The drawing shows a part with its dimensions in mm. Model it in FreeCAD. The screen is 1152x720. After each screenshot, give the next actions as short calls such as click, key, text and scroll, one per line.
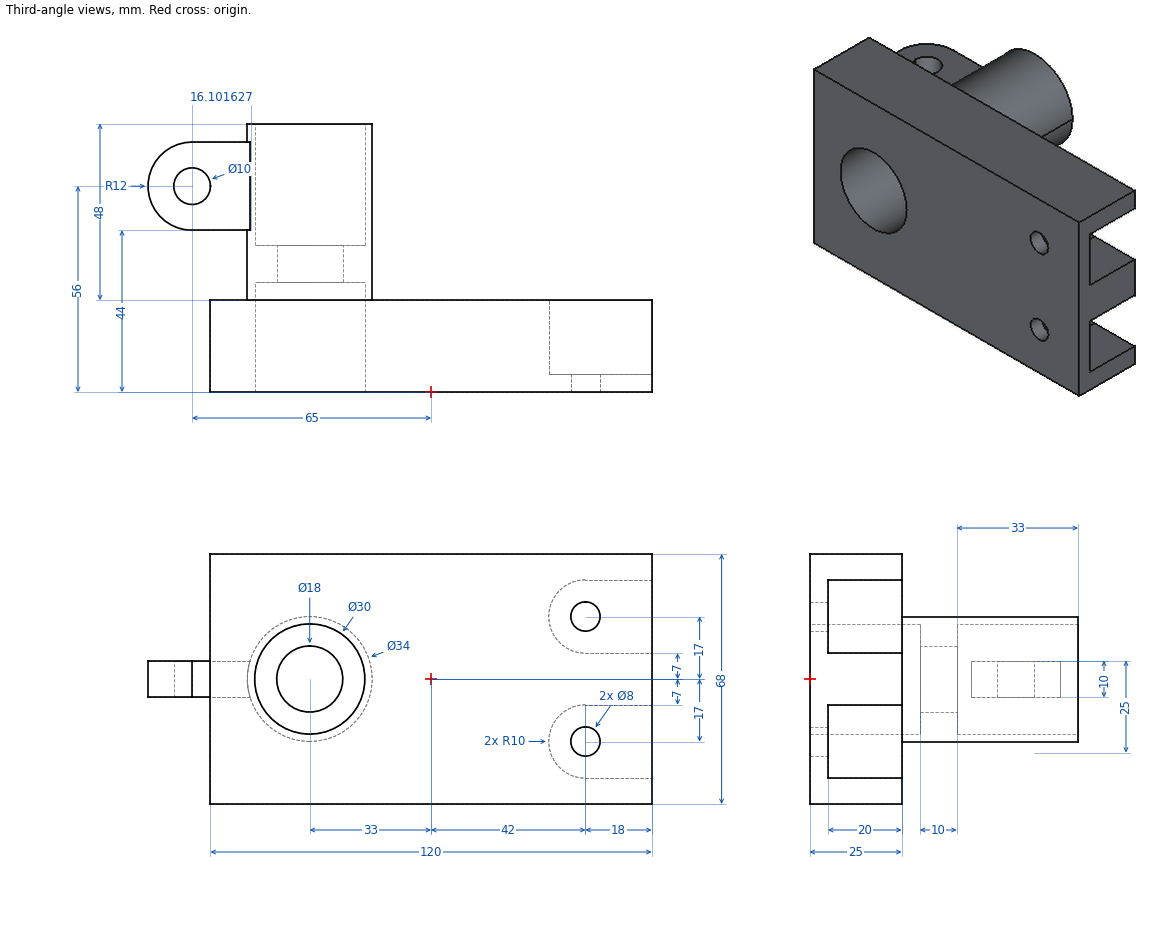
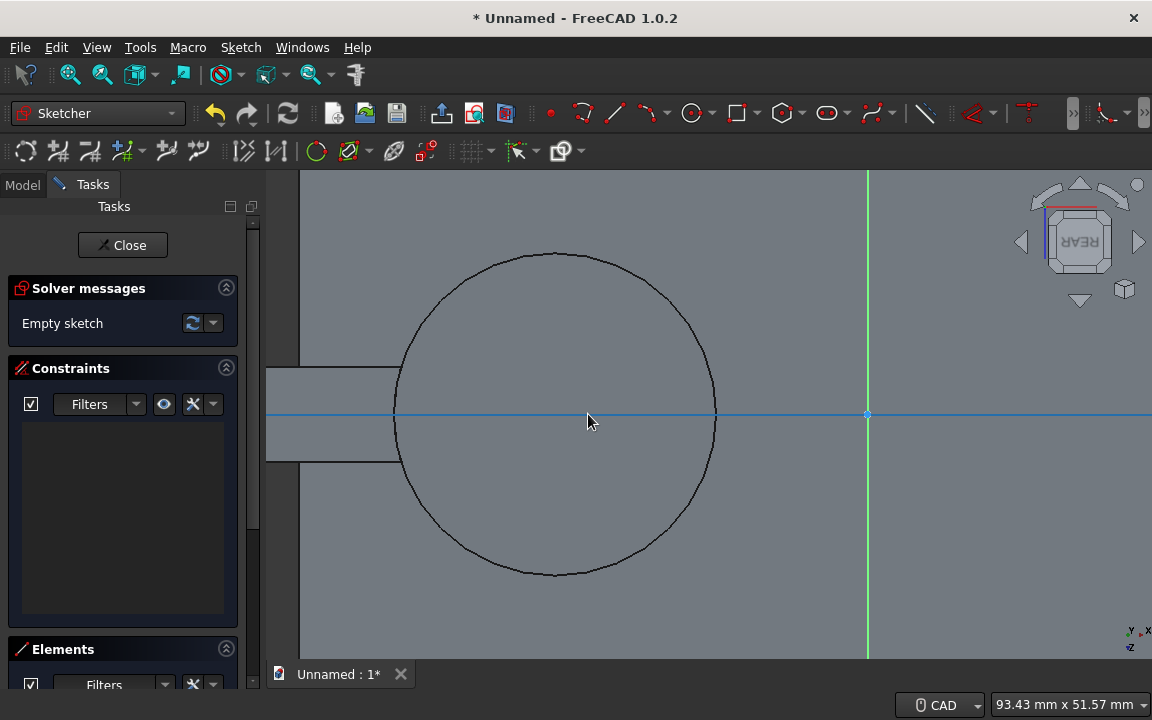
click(692, 114)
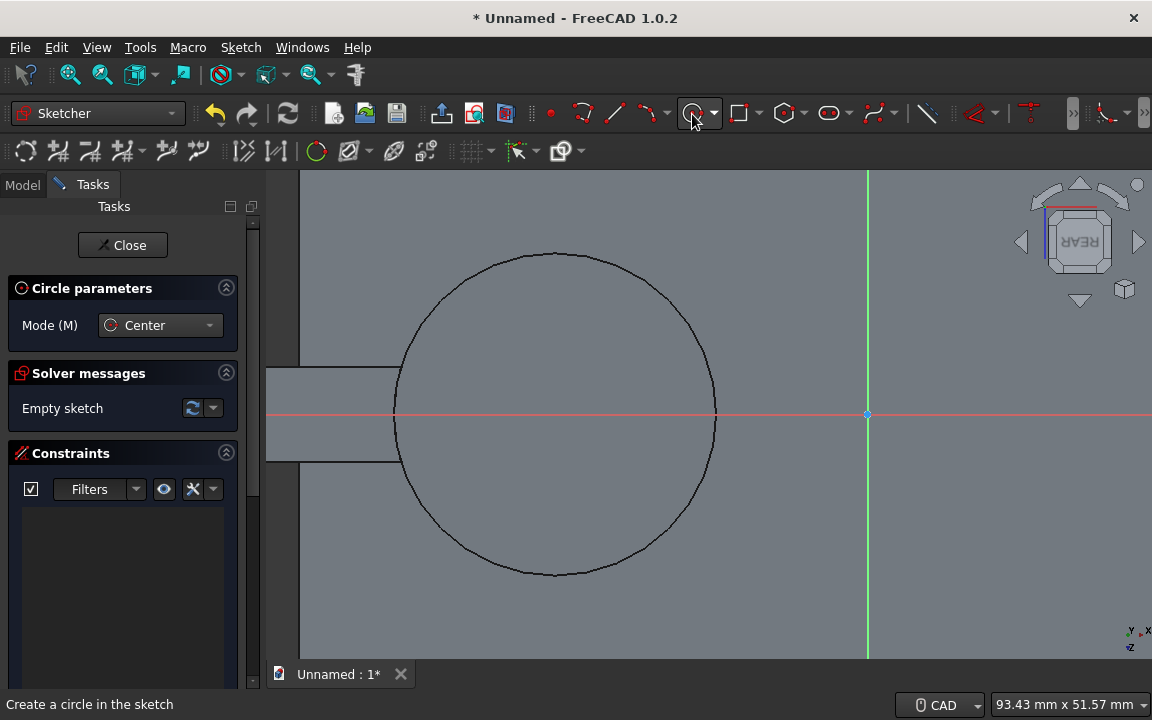
click(555, 414)
move(656, 314)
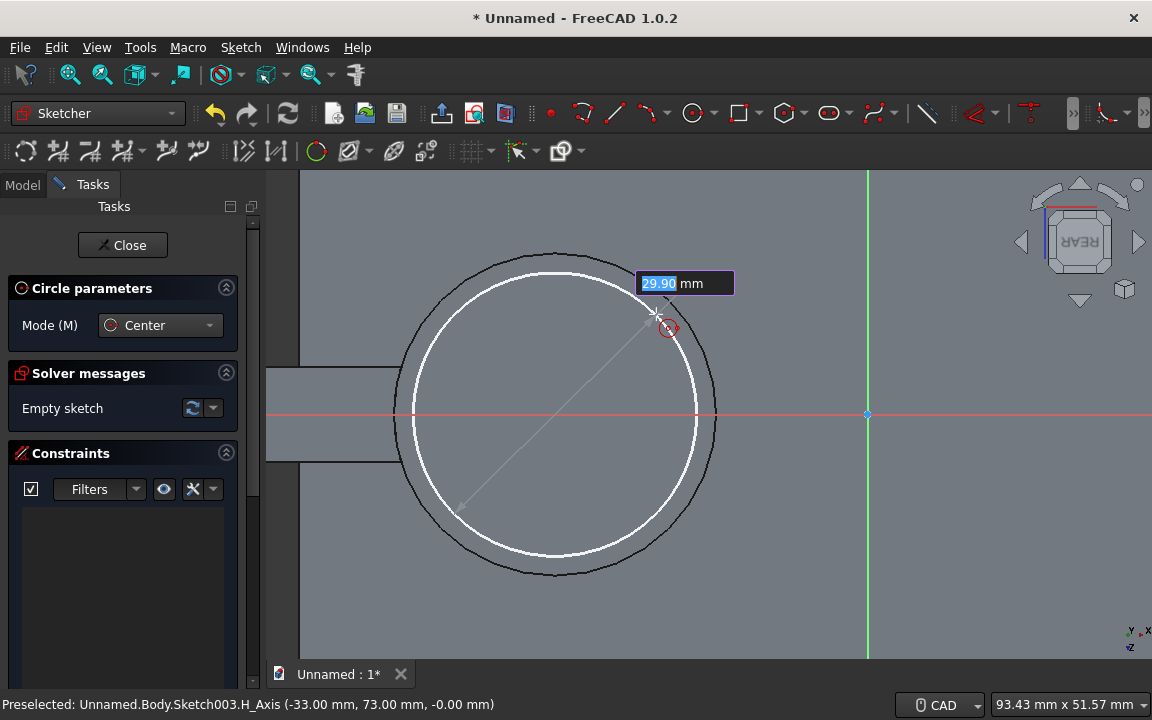
text(30)
key(Return)
key(Escape)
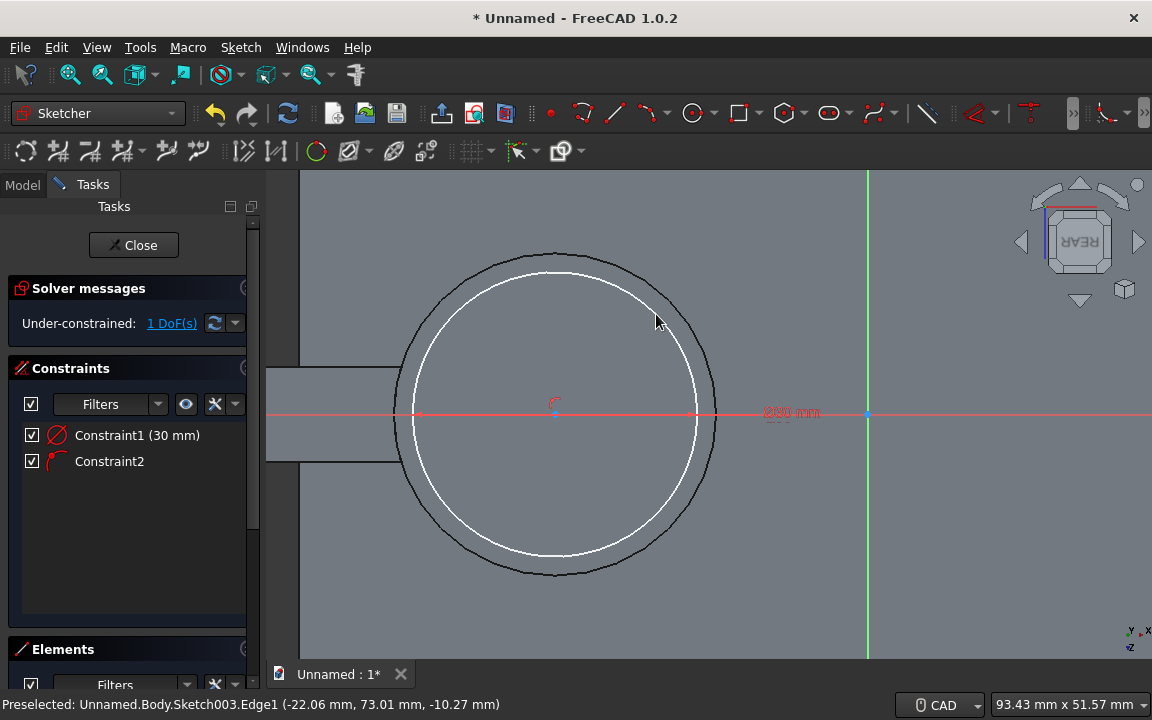
click(974, 114)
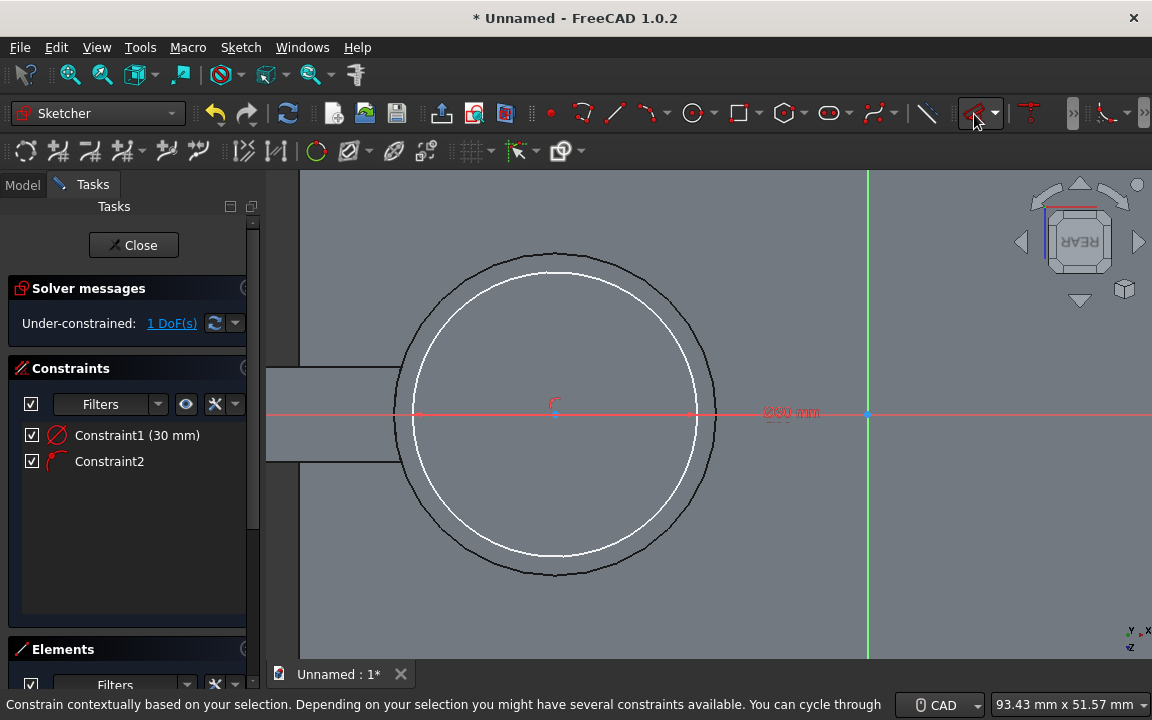
click(555, 414)
click(711, 448)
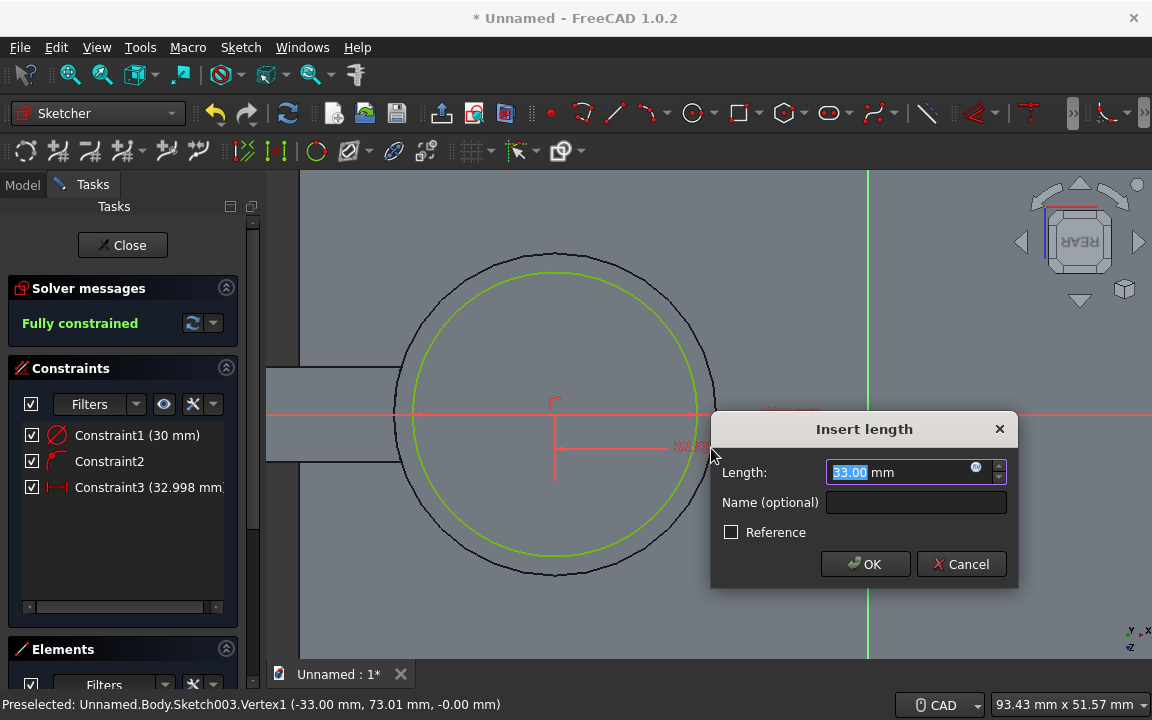
text(33)
key(Return)
key(Escape)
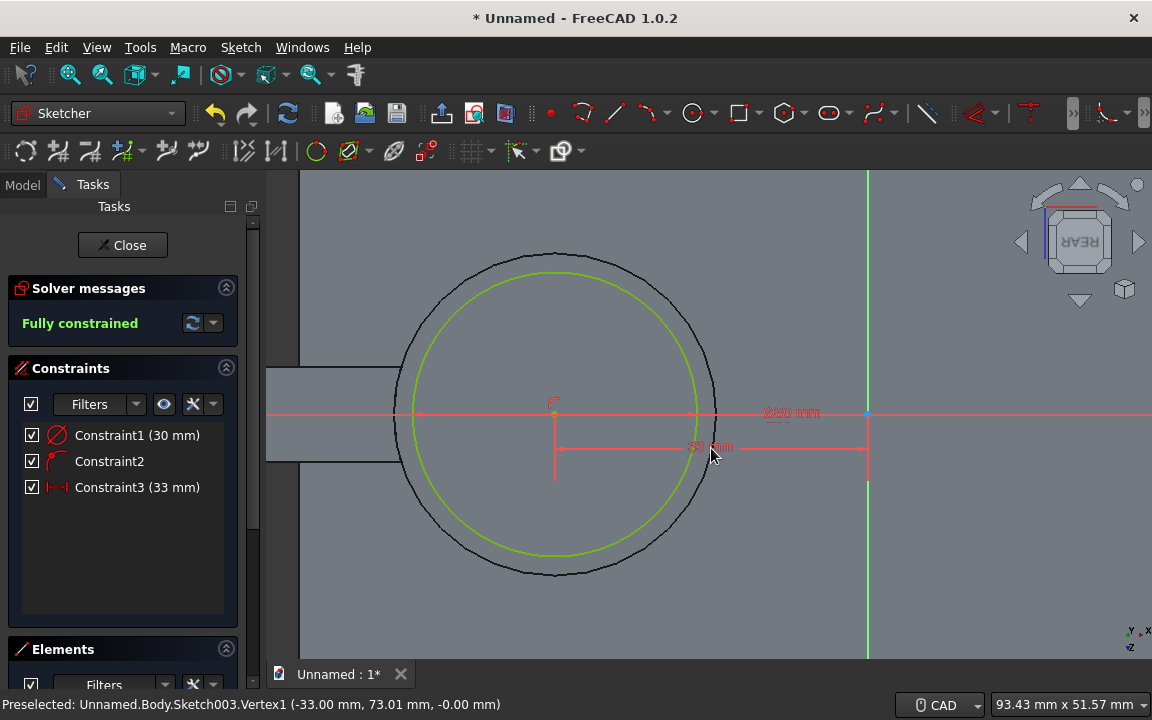
click(123, 245)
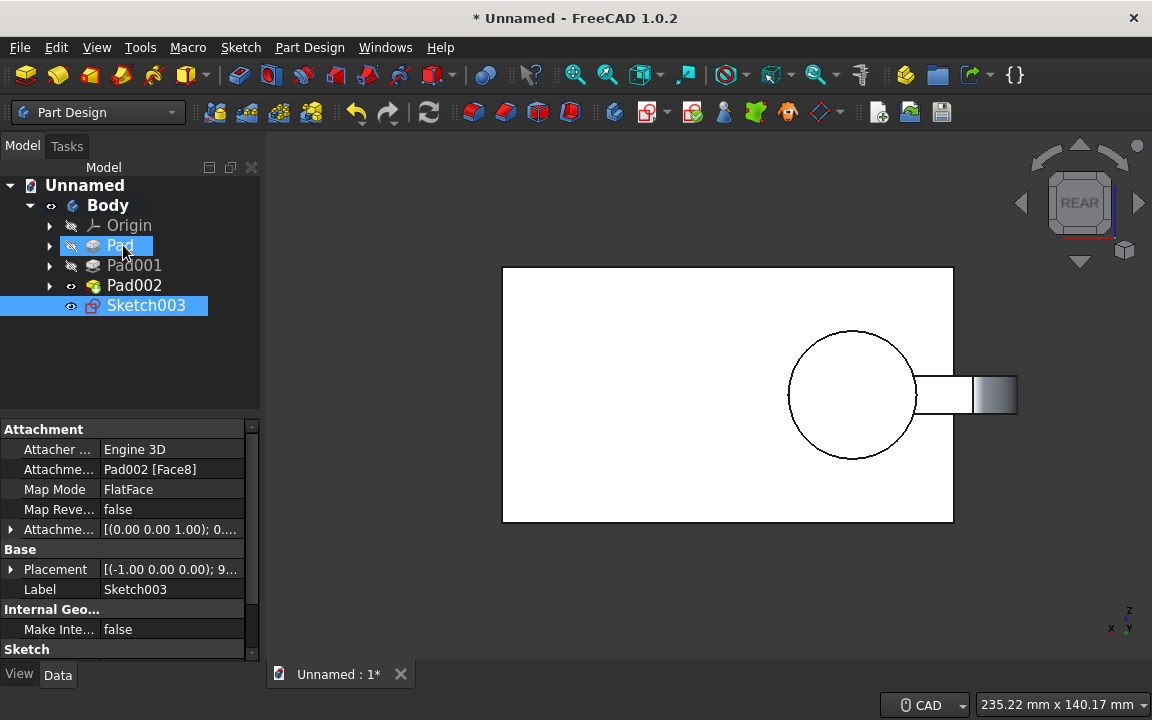
click(240, 76)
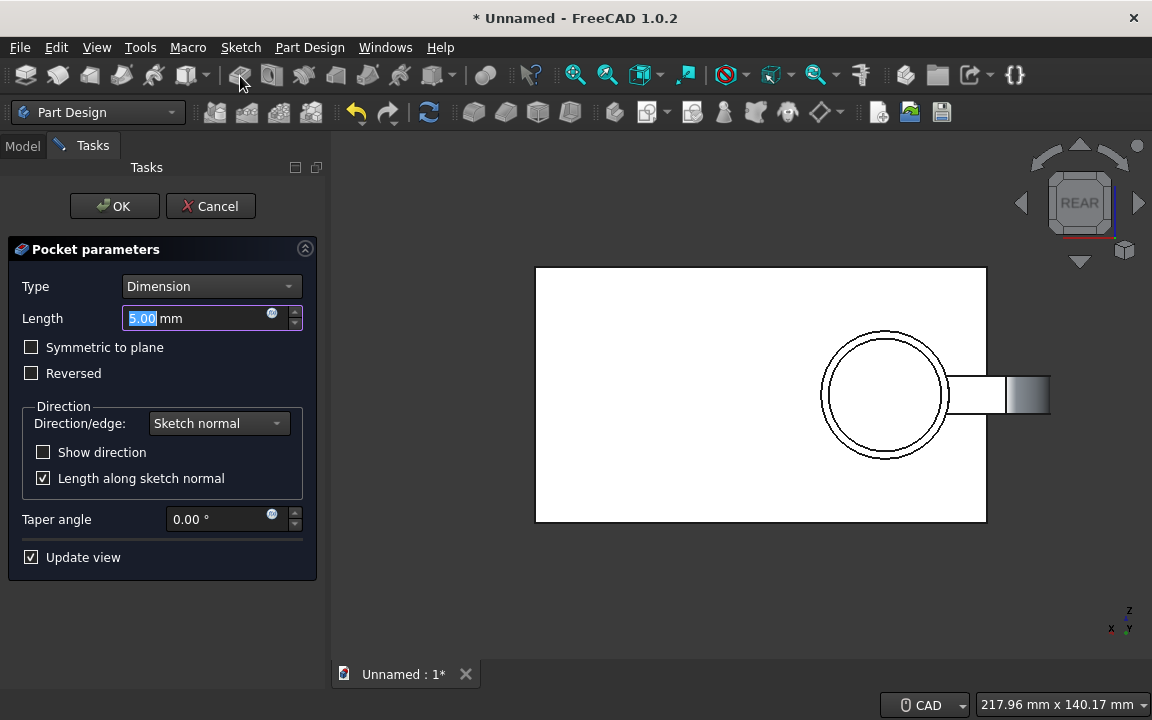
text(33)
key(Tab)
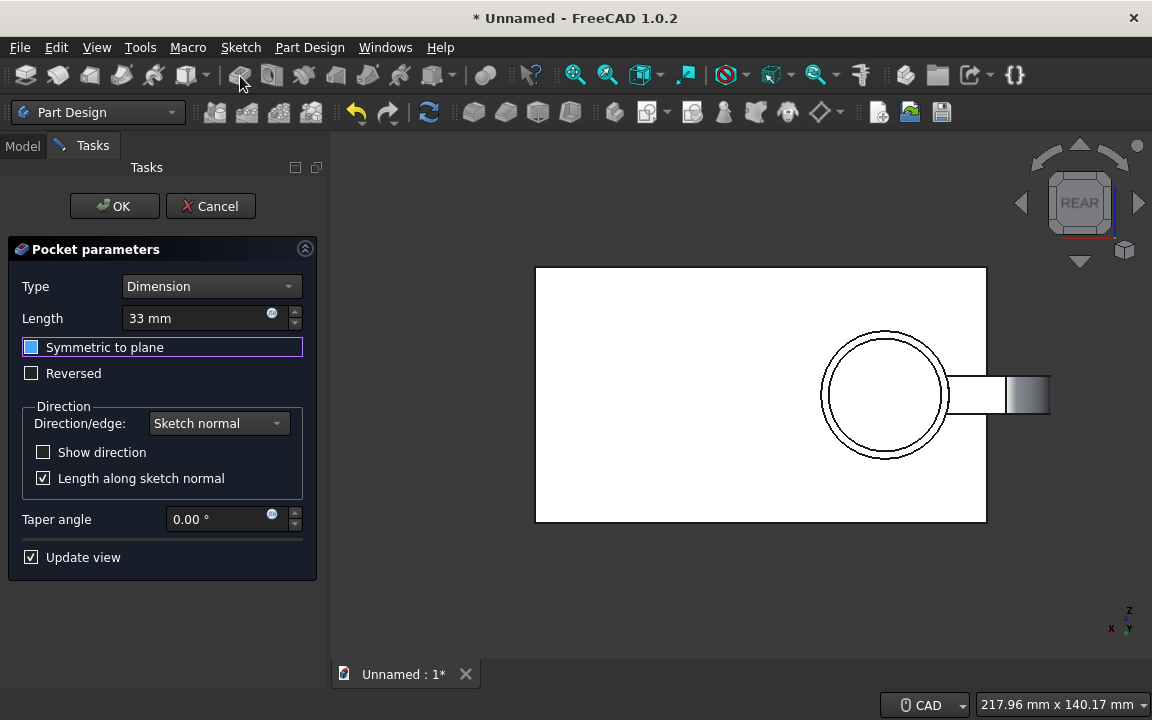
click(115, 206)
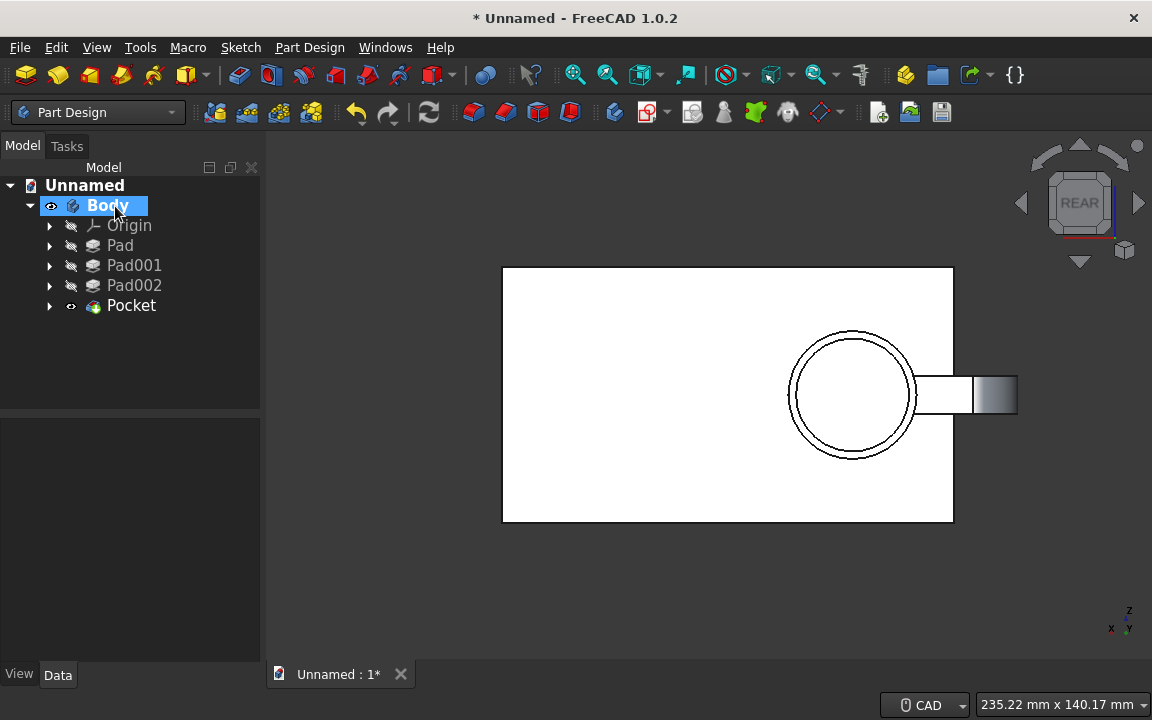
click(853, 394)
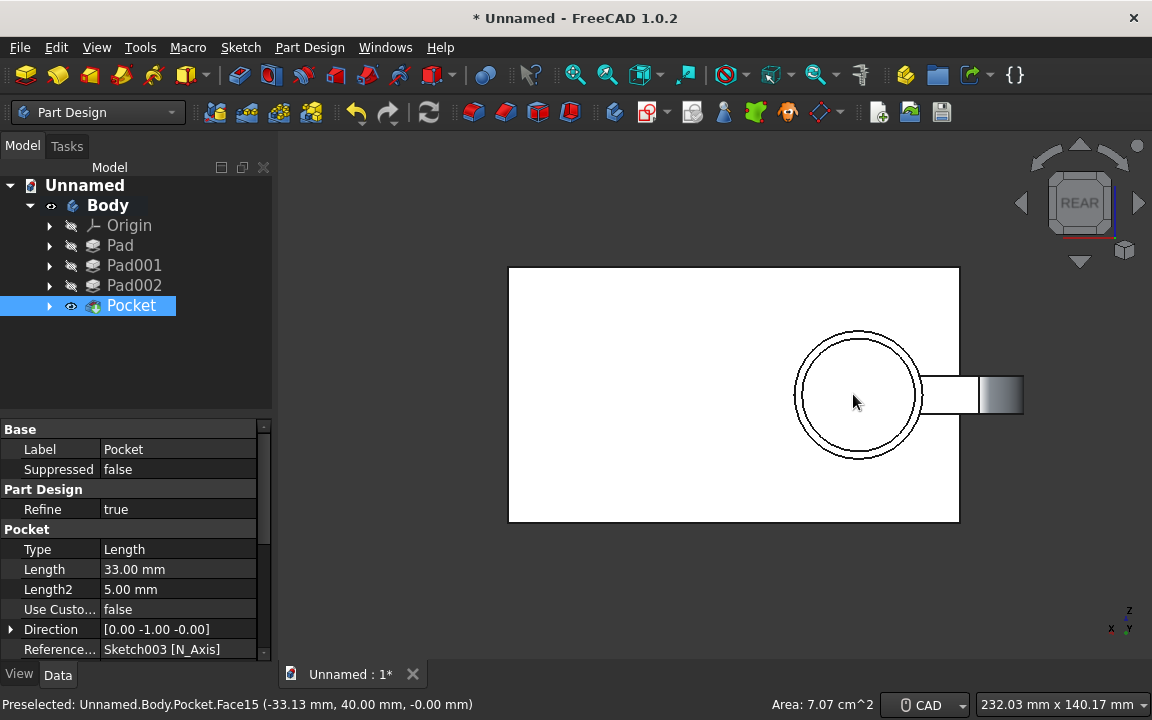
click(648, 112)